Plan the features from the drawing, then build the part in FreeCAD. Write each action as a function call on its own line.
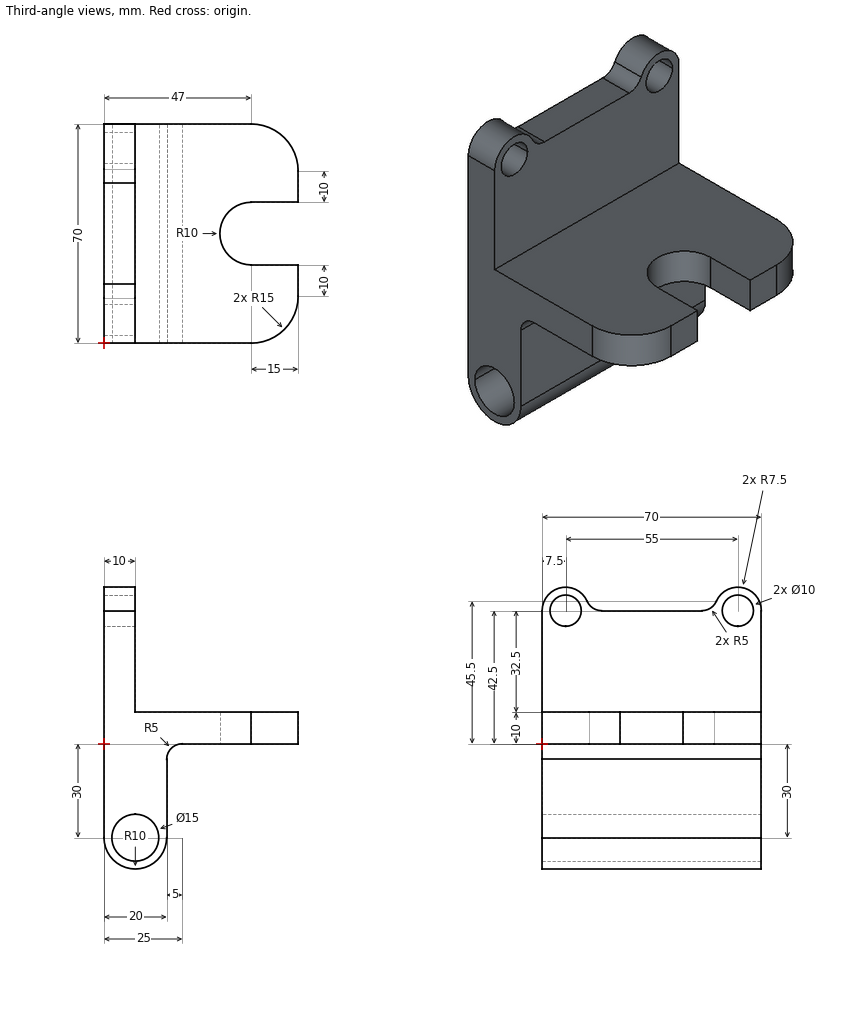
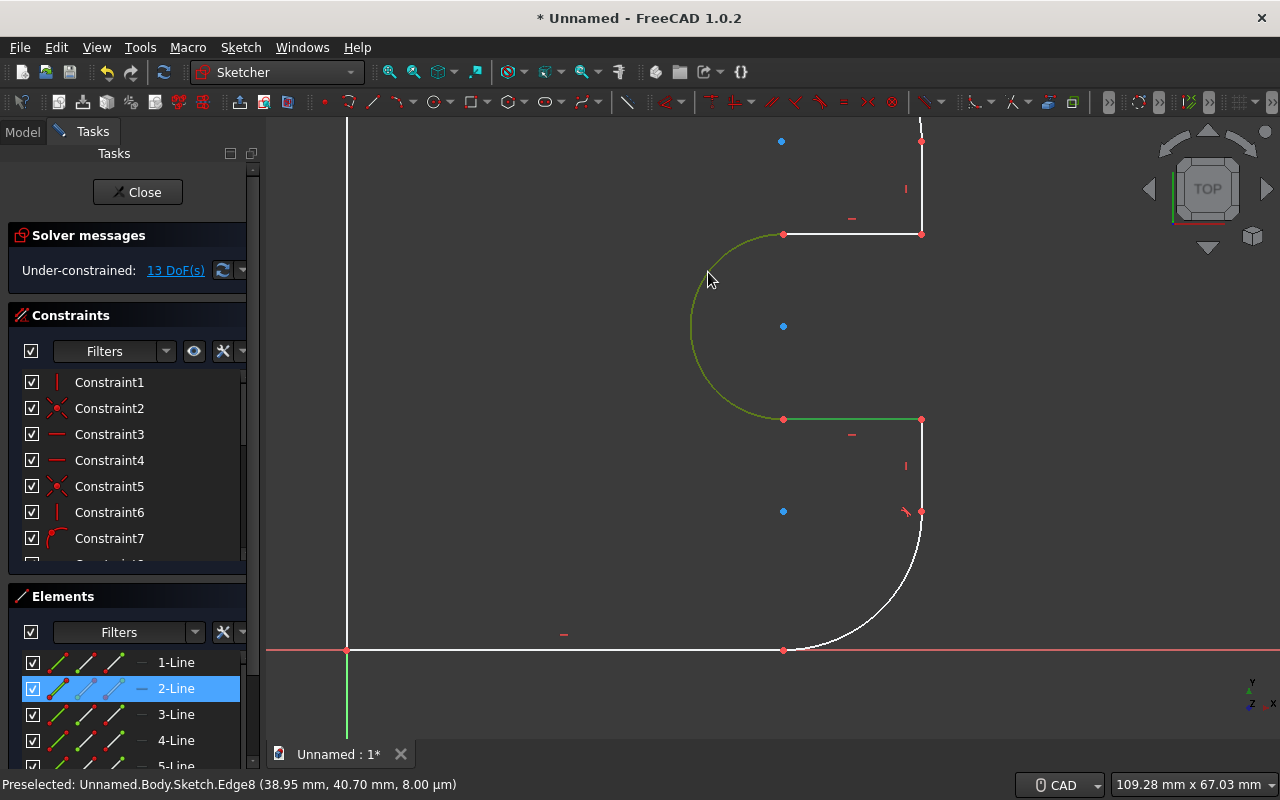
click(820, 102)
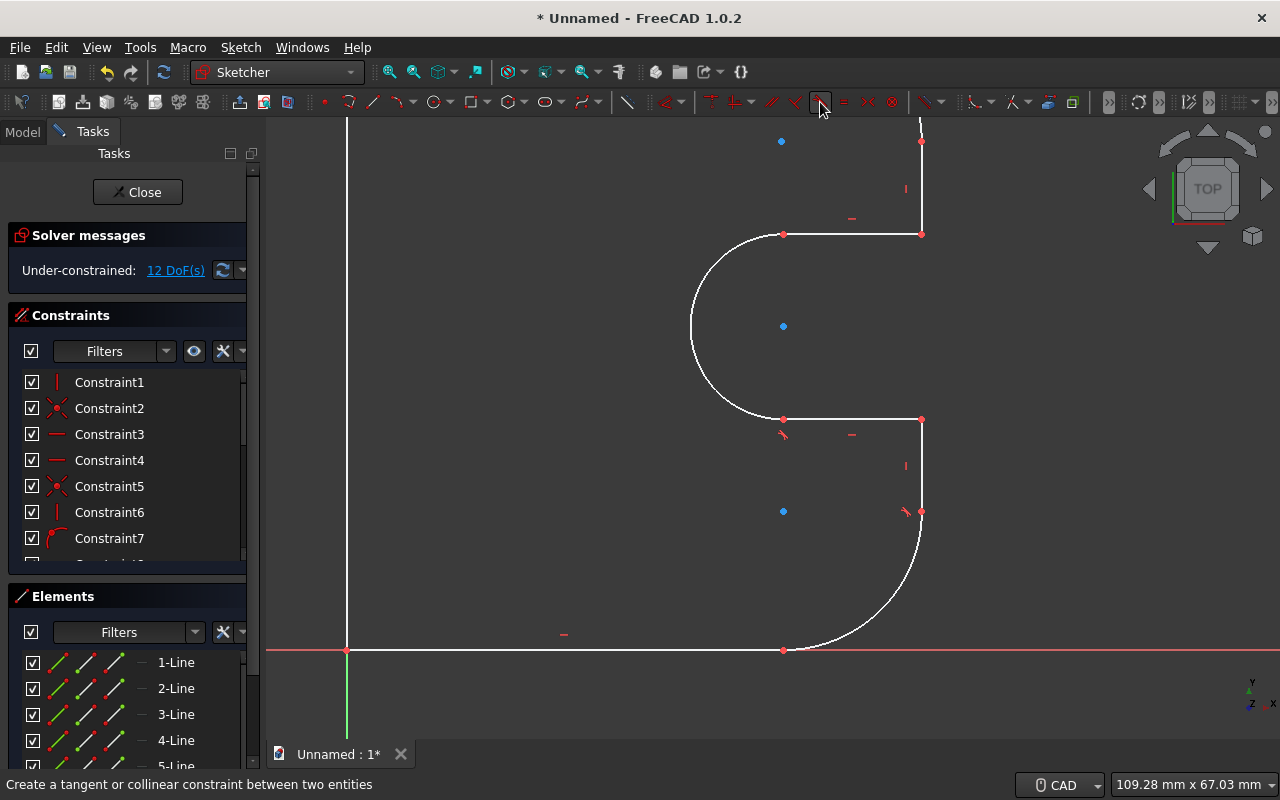
click(825, 234)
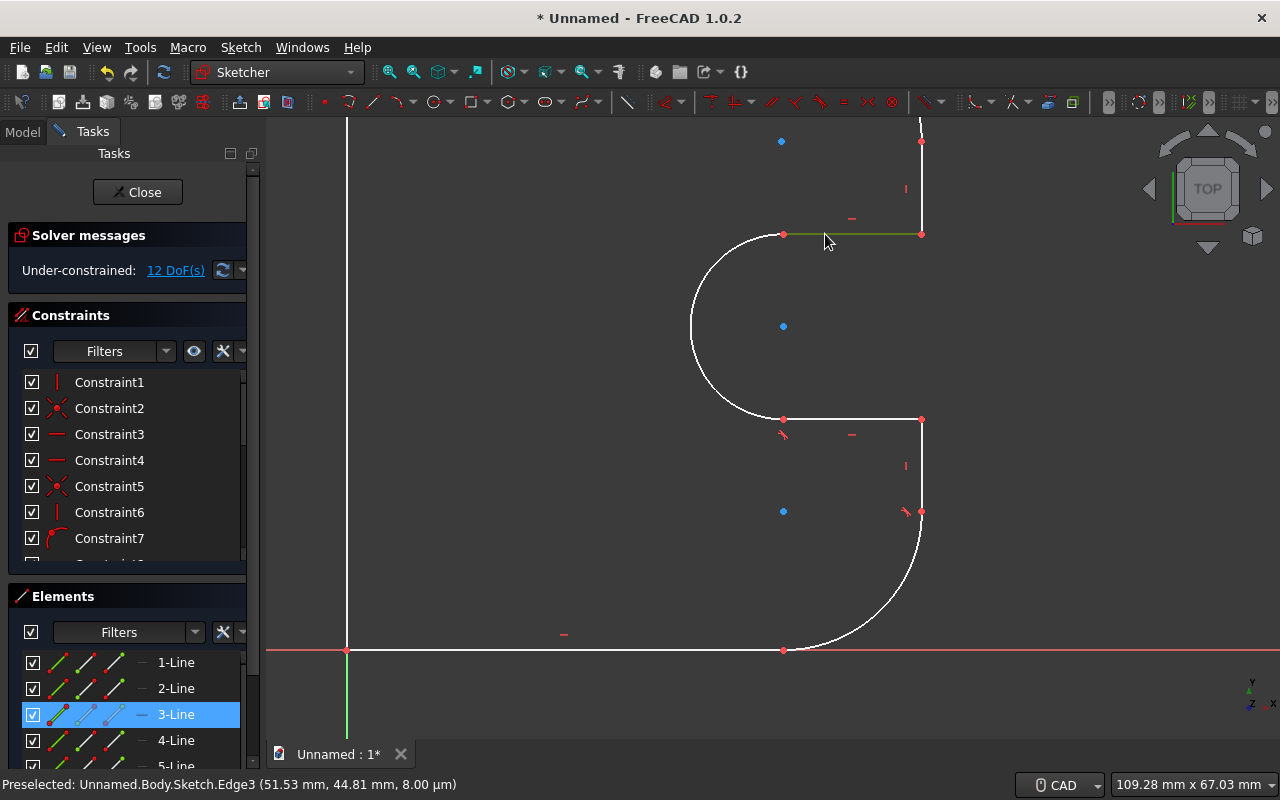
click(708, 272)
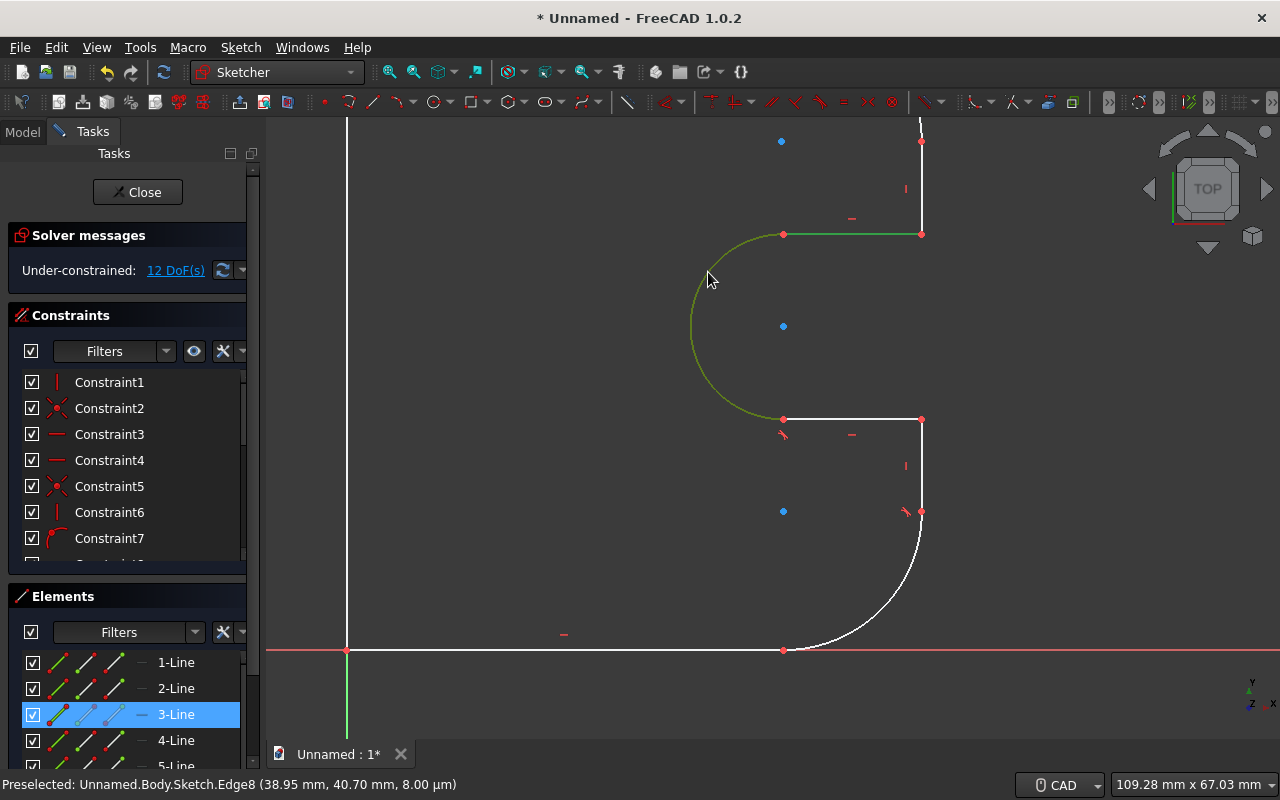
click(820, 102)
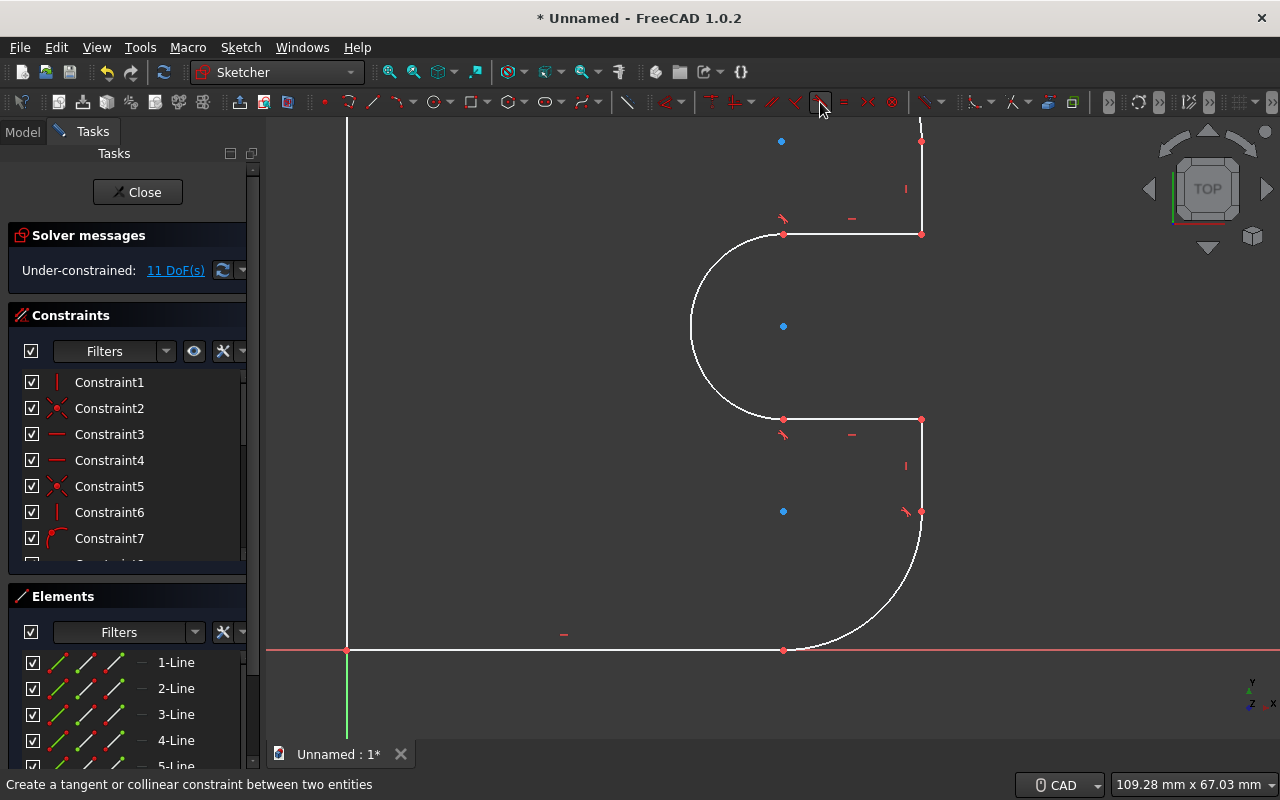
click(922, 207)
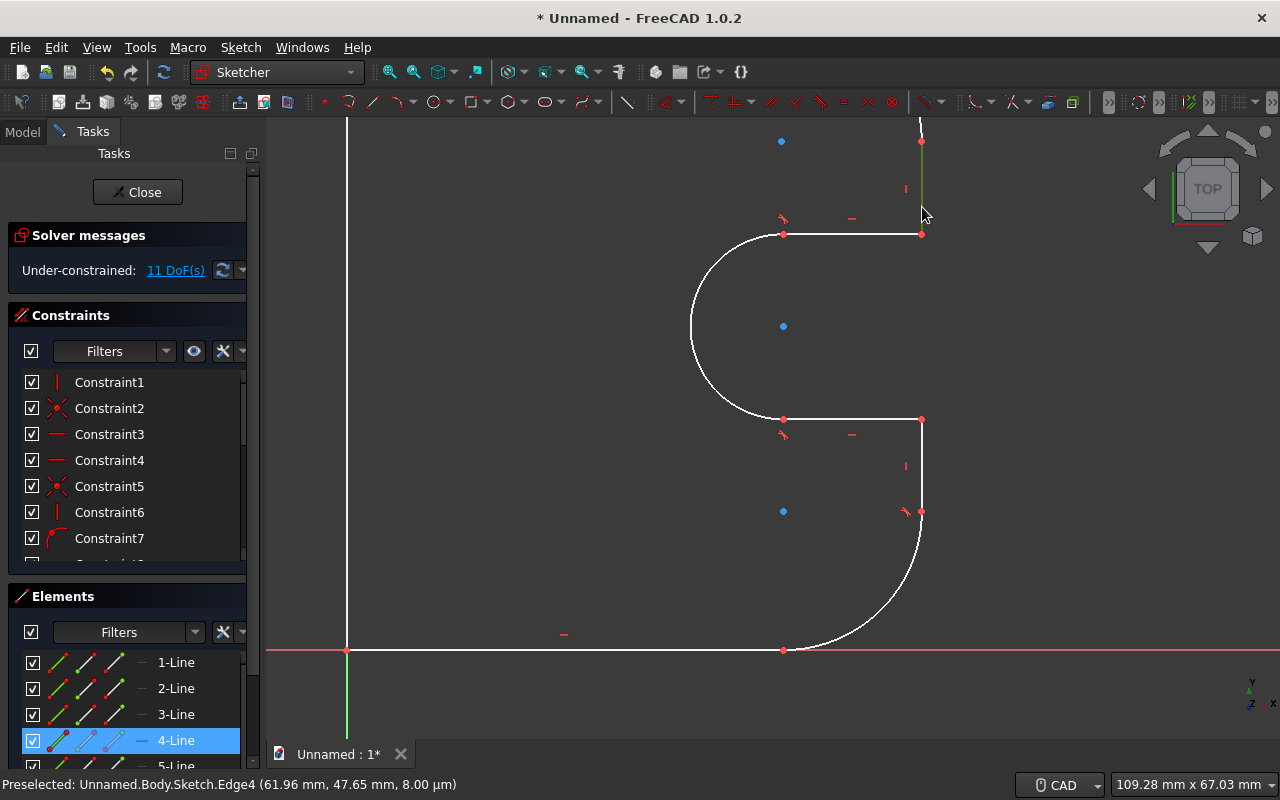
scroll(847, 637, down, 2)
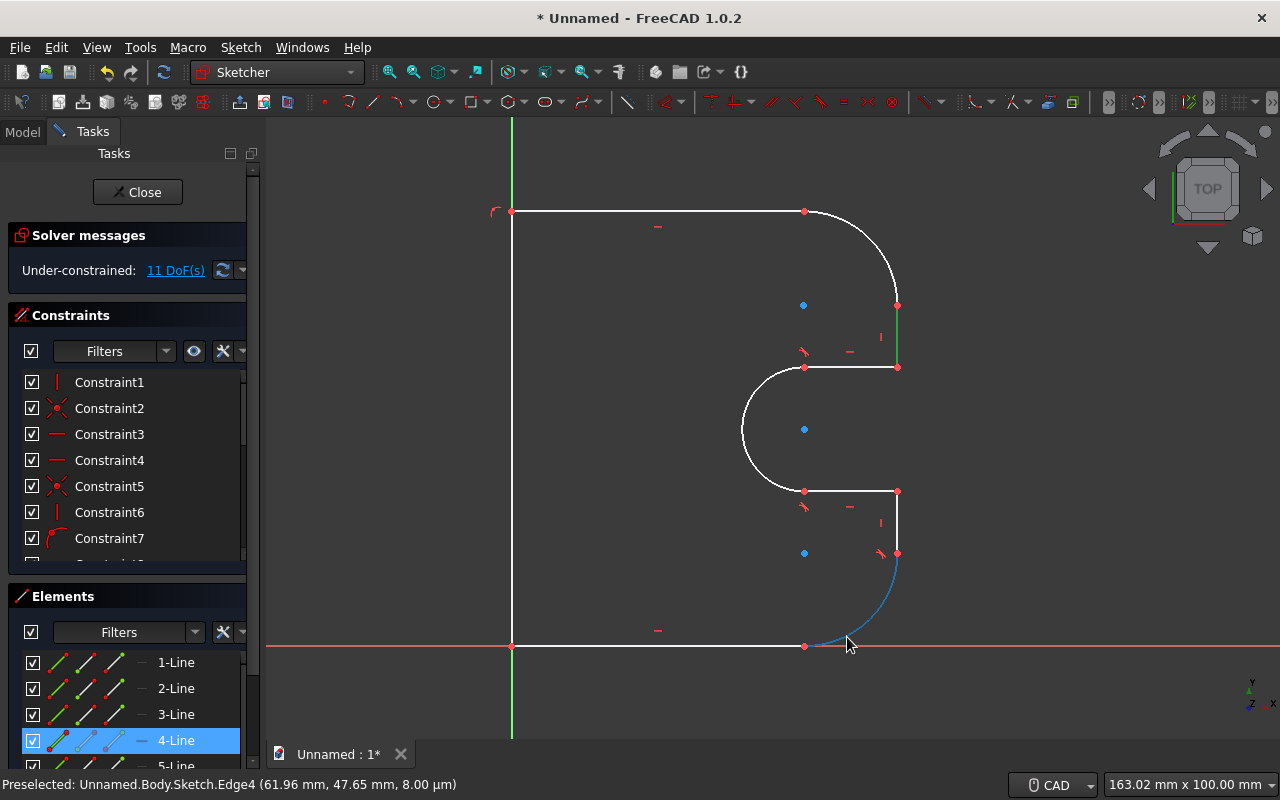
click(887, 263)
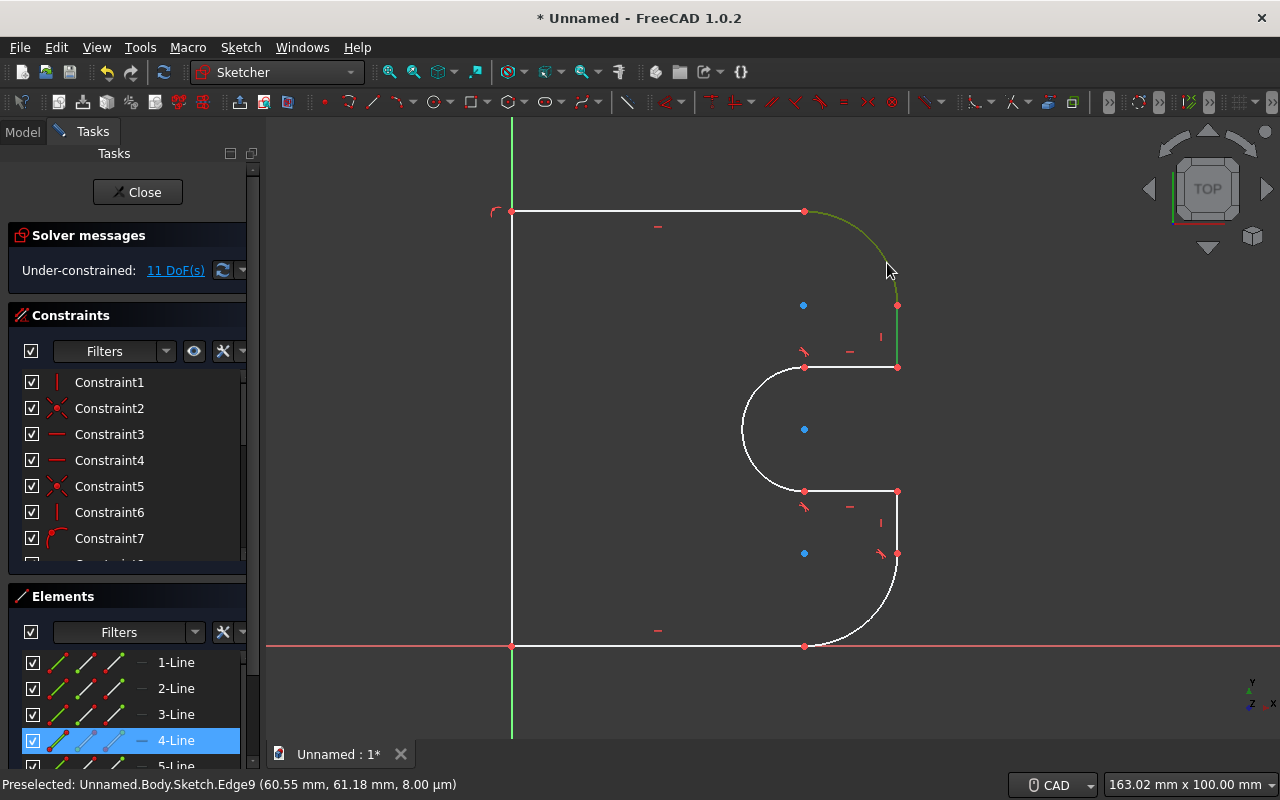
click(820, 102)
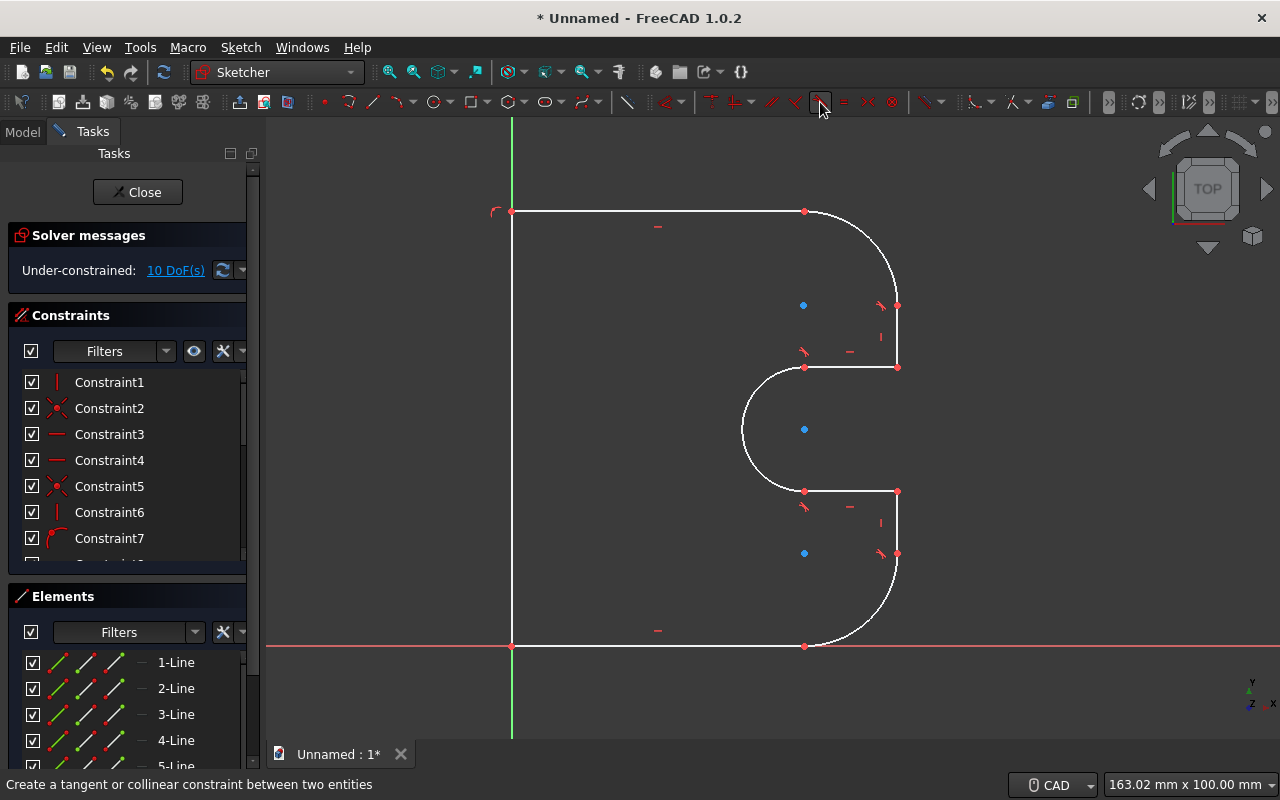
click(717, 211)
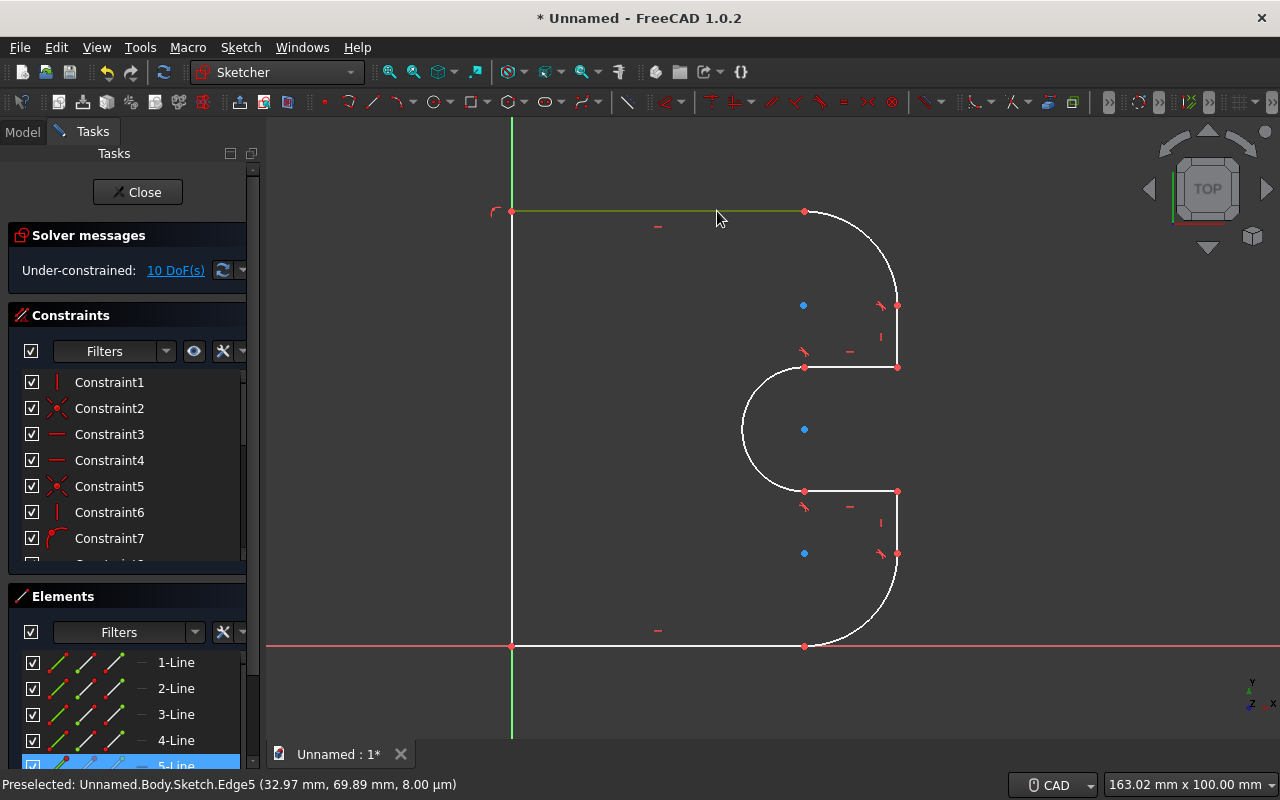
click(887, 263)